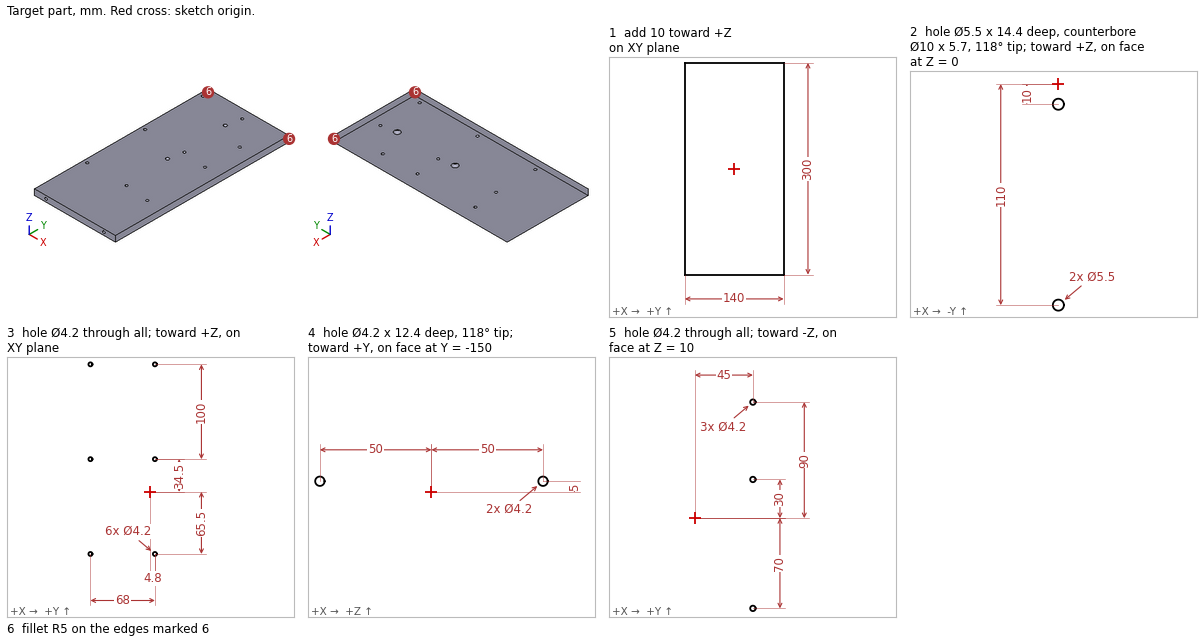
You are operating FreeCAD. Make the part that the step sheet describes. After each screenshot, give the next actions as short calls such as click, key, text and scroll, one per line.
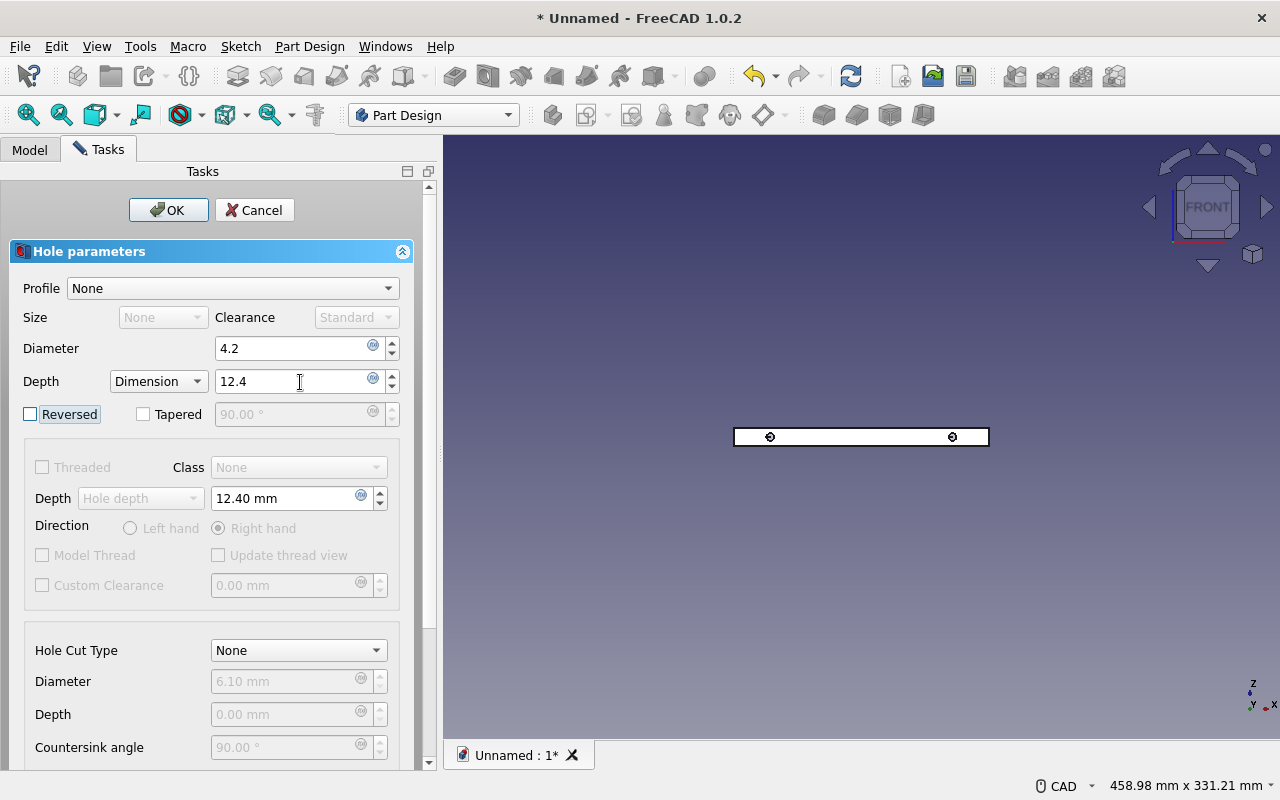
click(169, 210)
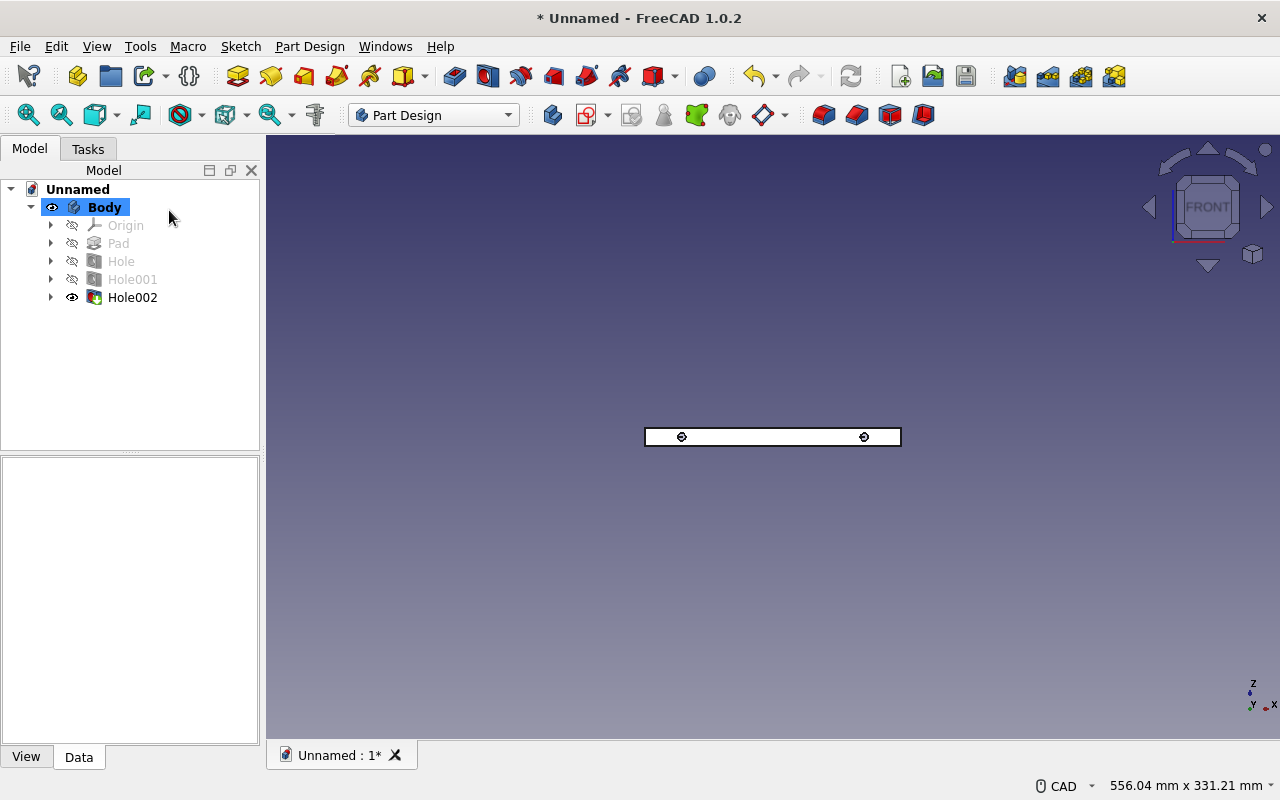
key(v)
key(f)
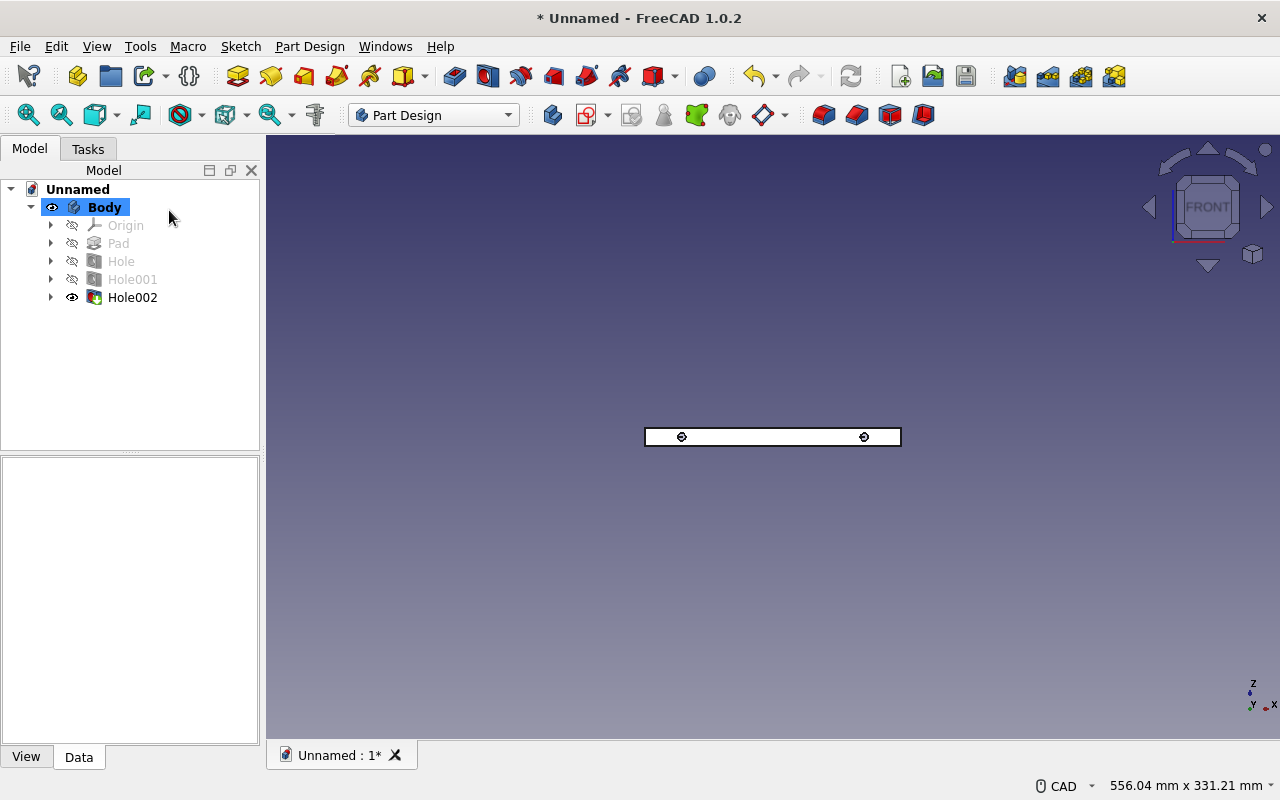
key(0)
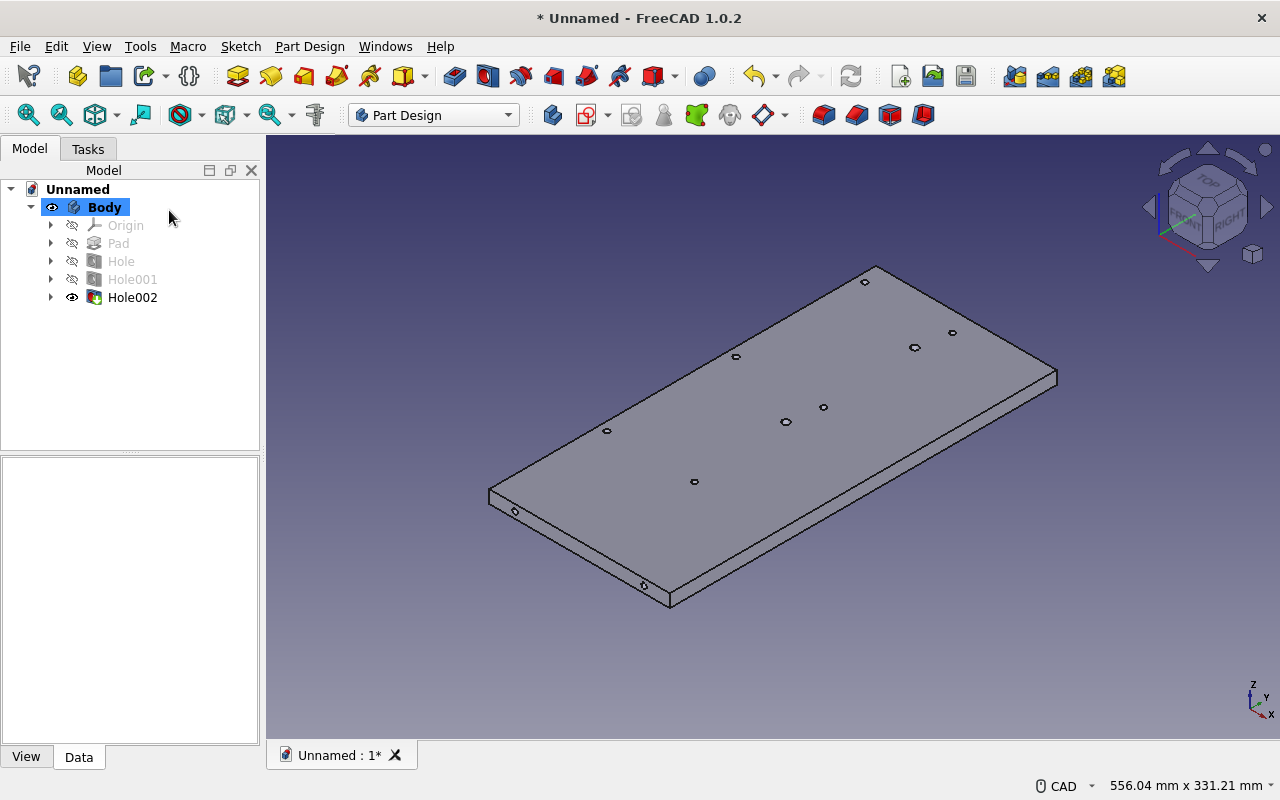
click(692, 446)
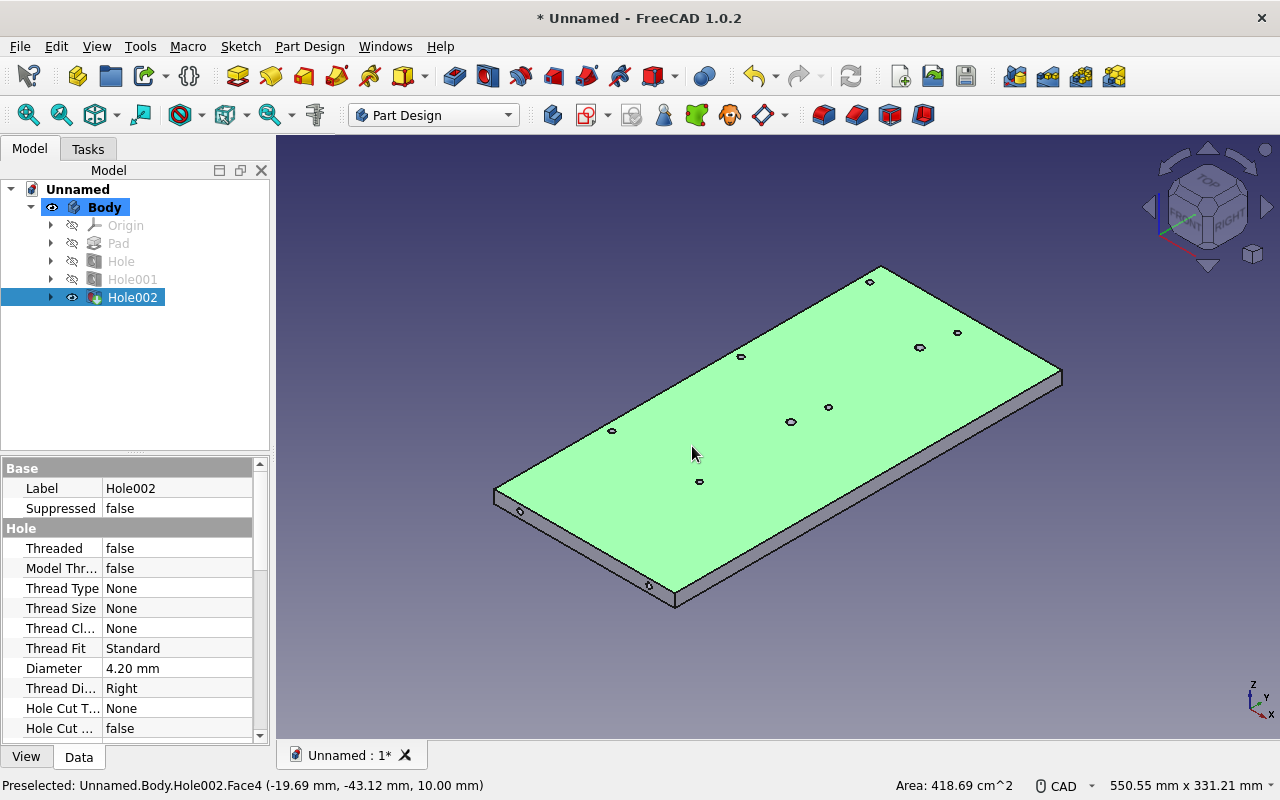
click(586, 116)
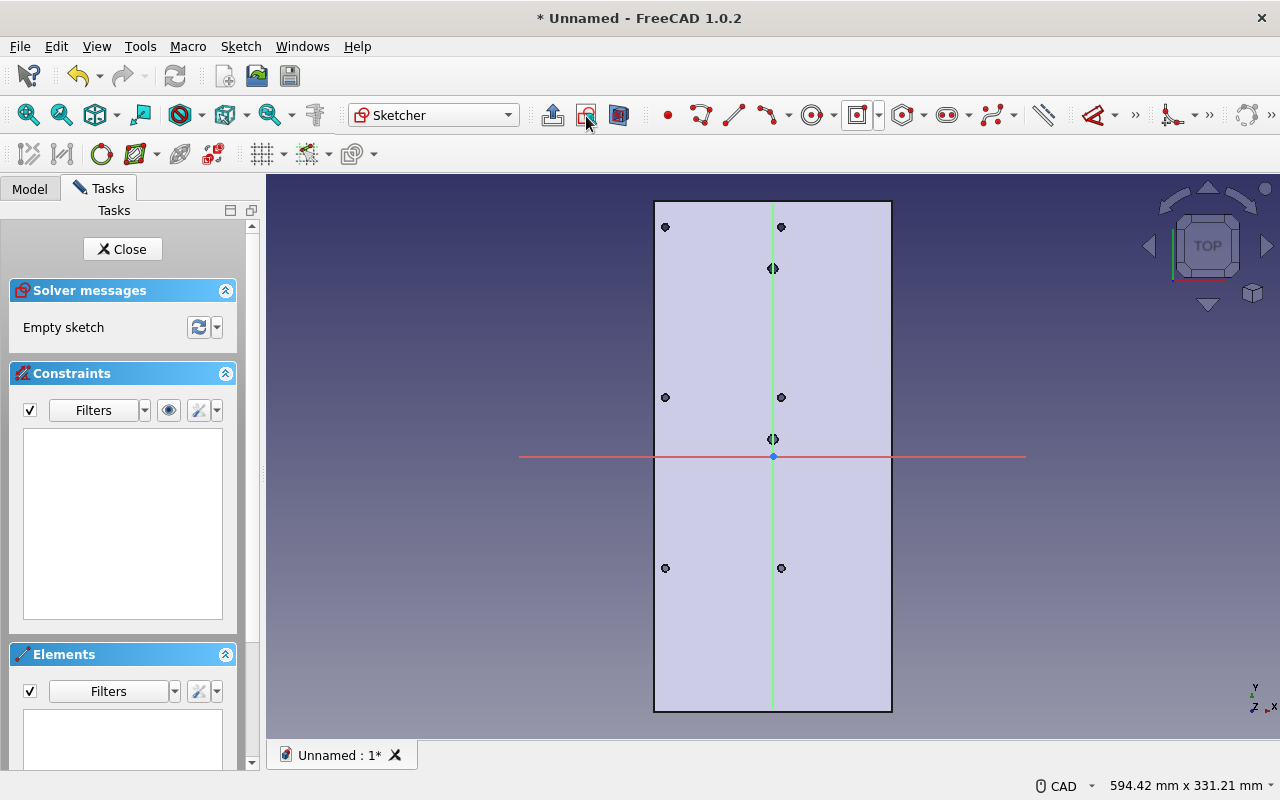
key(g)
key(c)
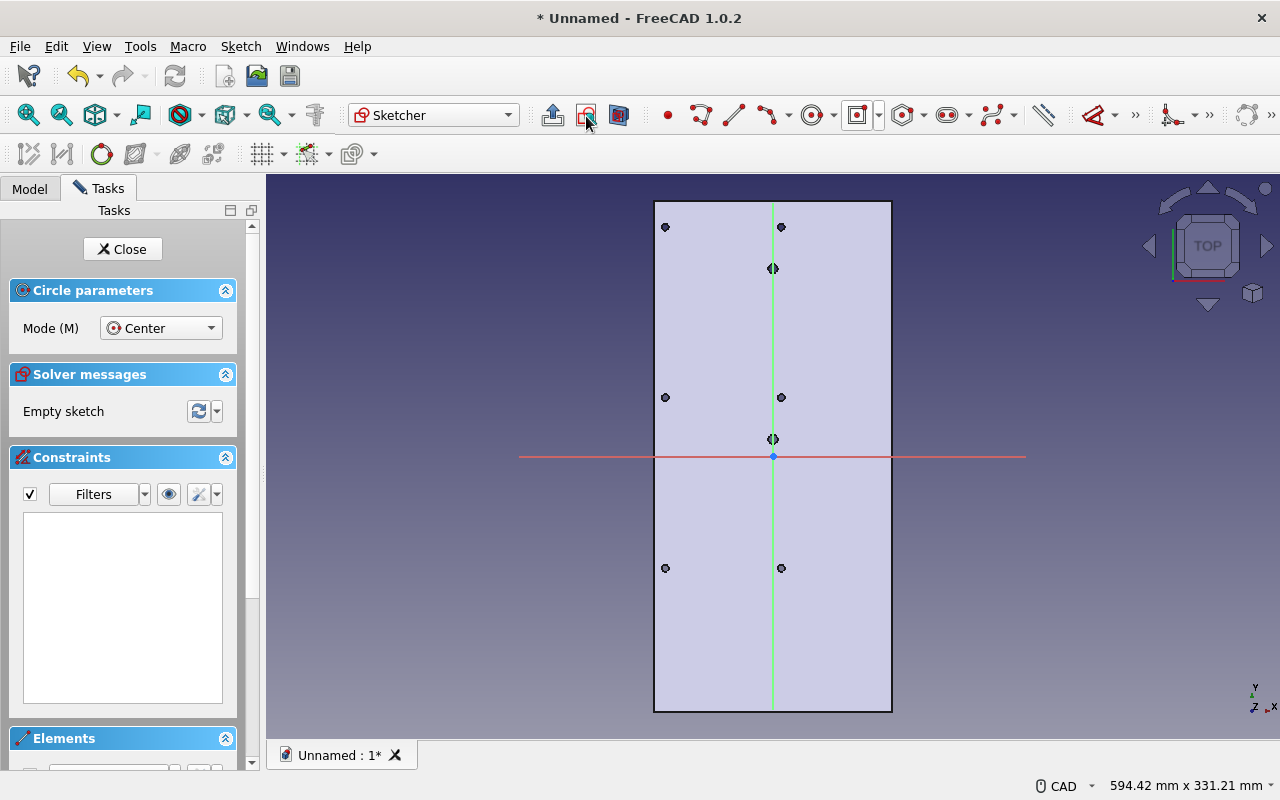
scroll(850, 303, up, 10)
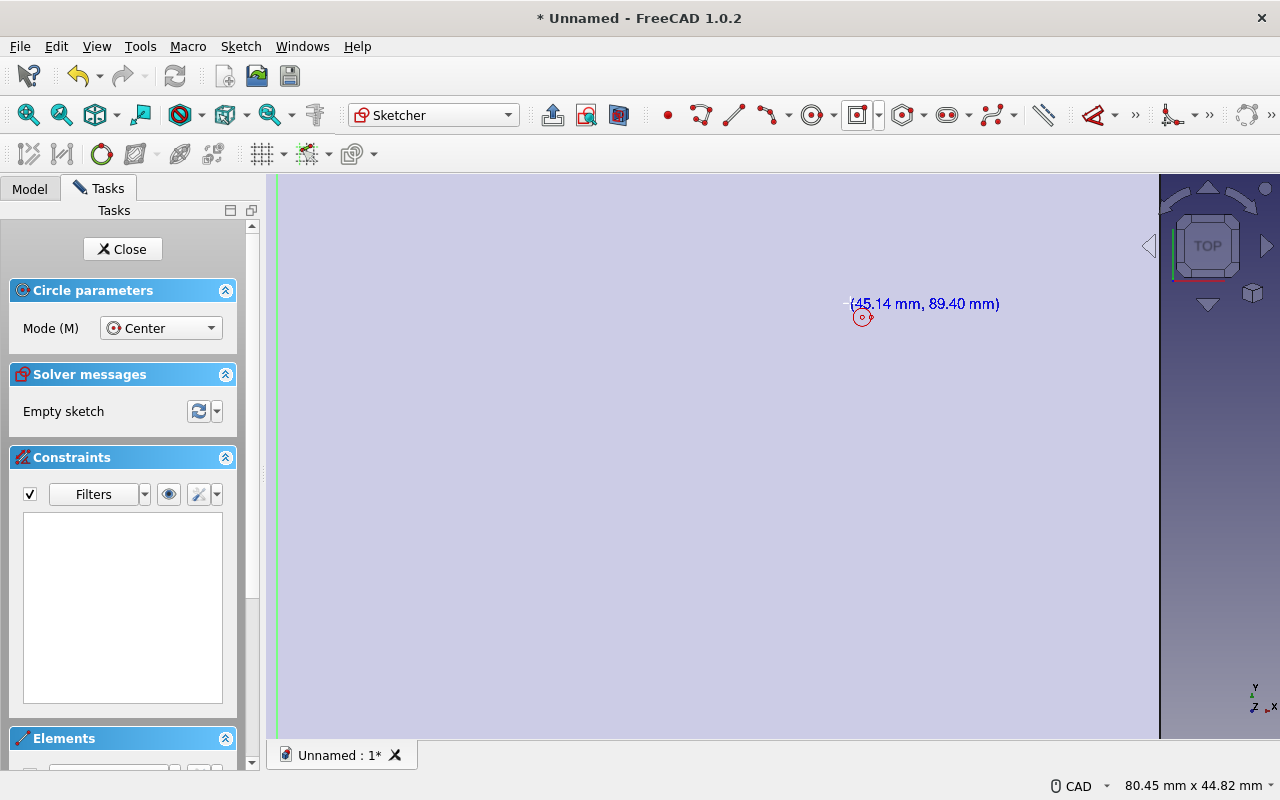
scroll(730, 288, down, 9)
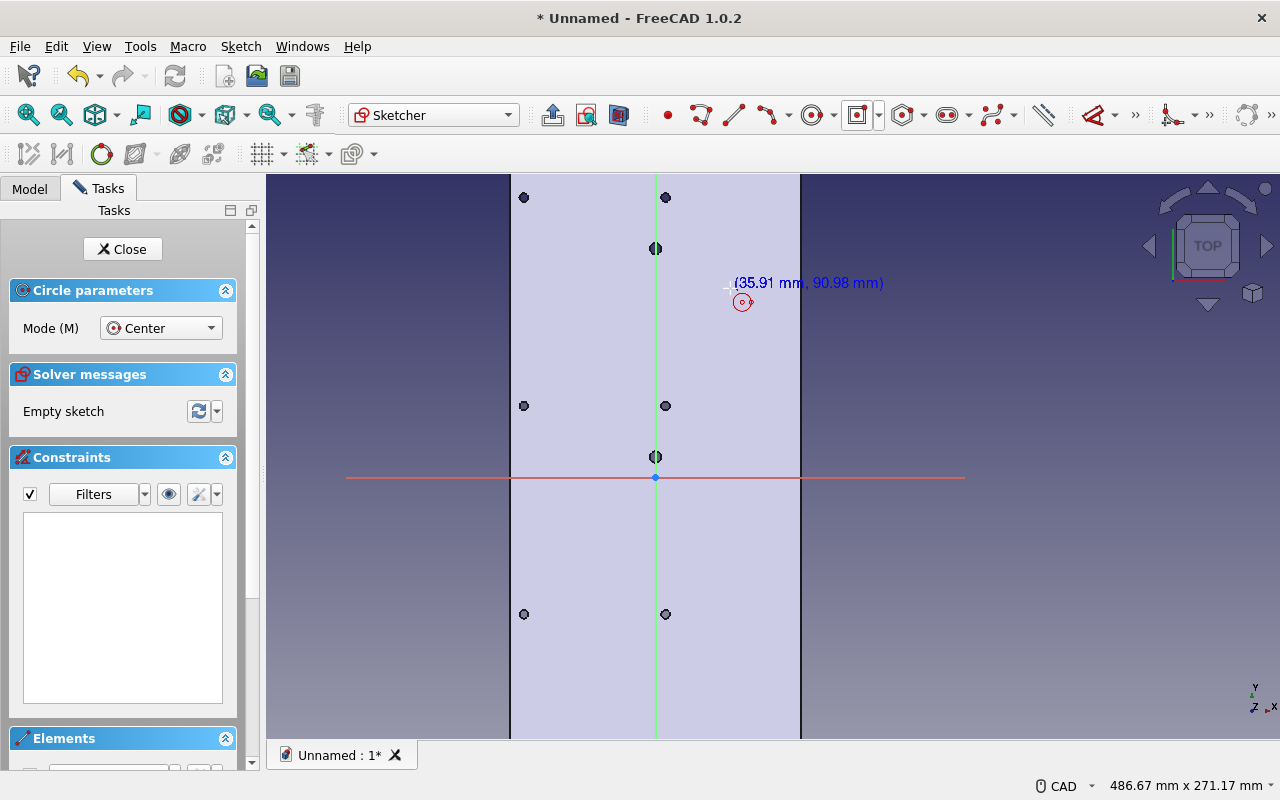
click(749, 290)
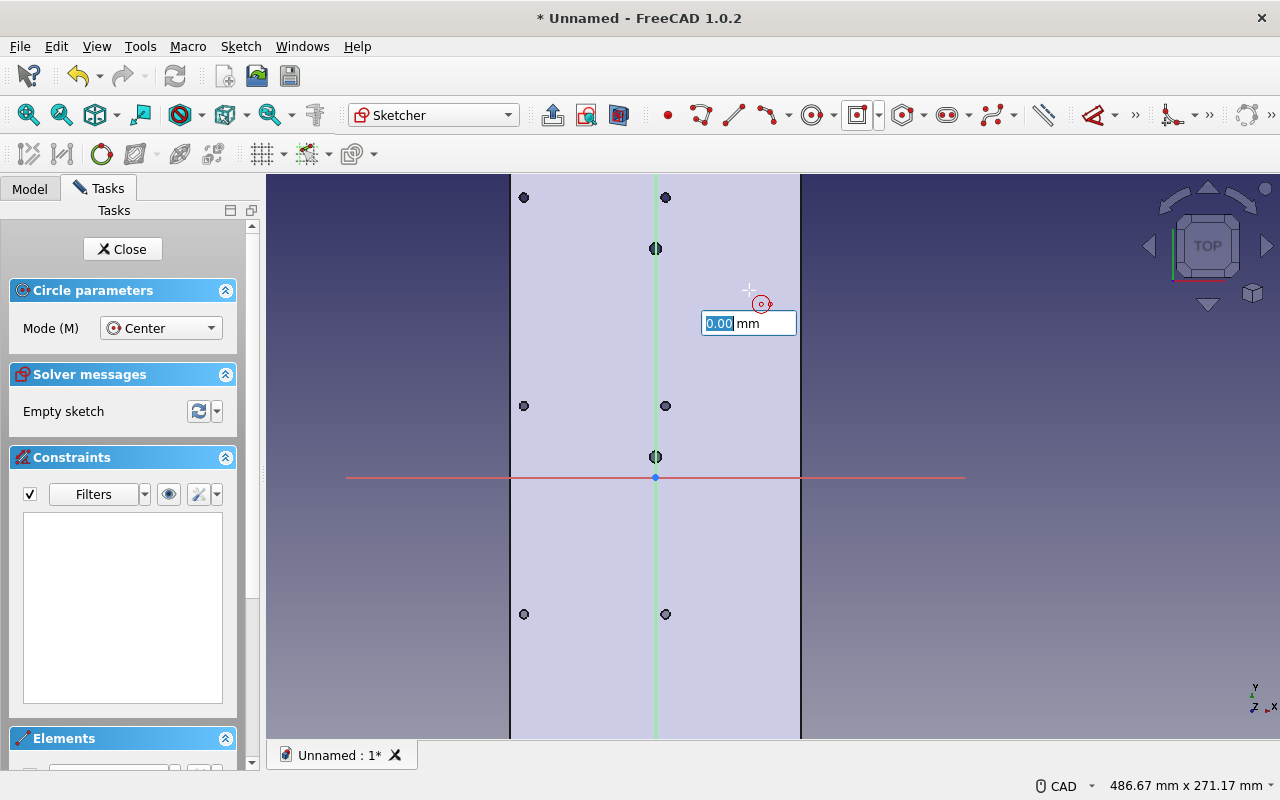
scroll(752, 287, up, 7)